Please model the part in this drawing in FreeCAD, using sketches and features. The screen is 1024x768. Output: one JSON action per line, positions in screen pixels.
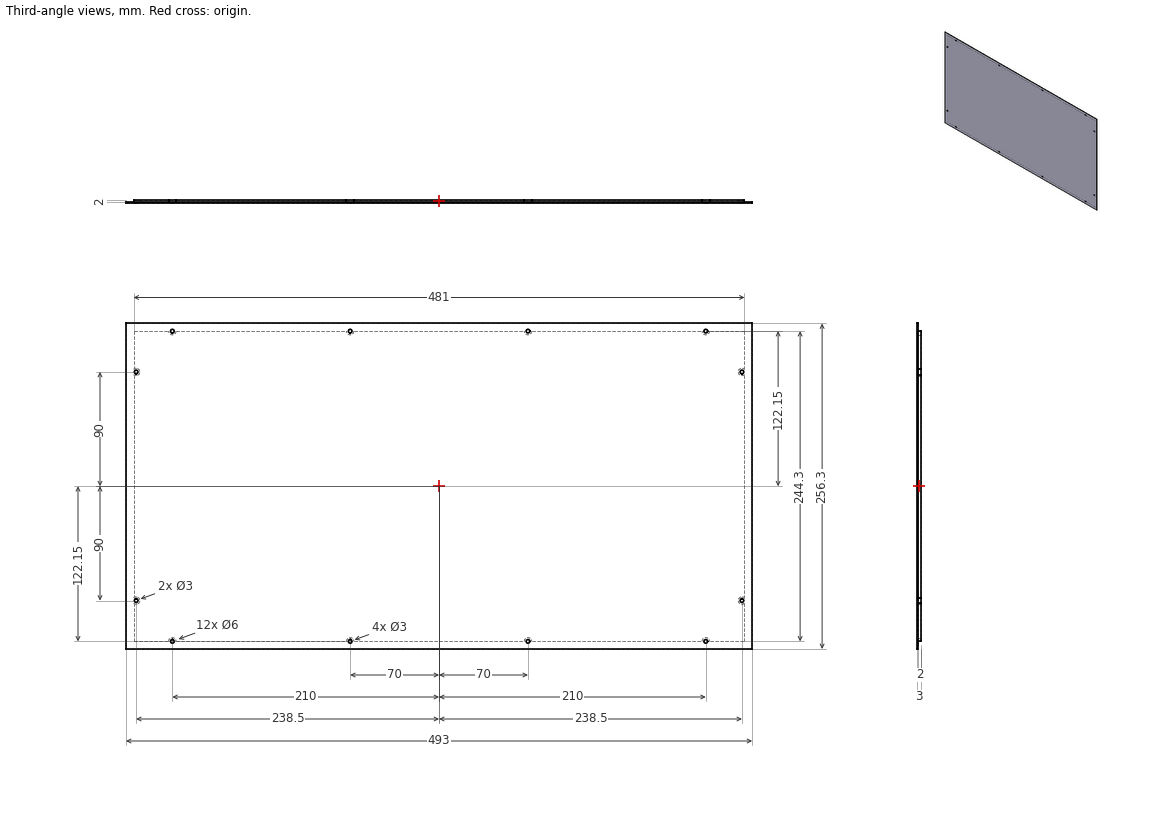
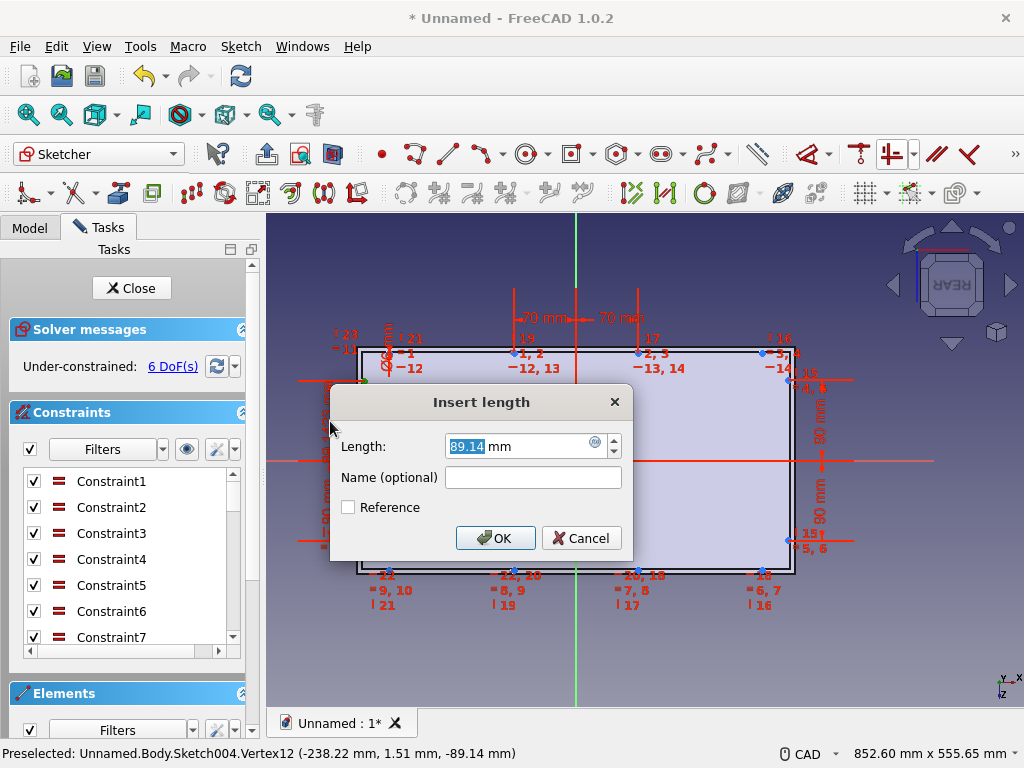
{"action": "type", "text": "90"}
{"action": "key", "text": "Return"}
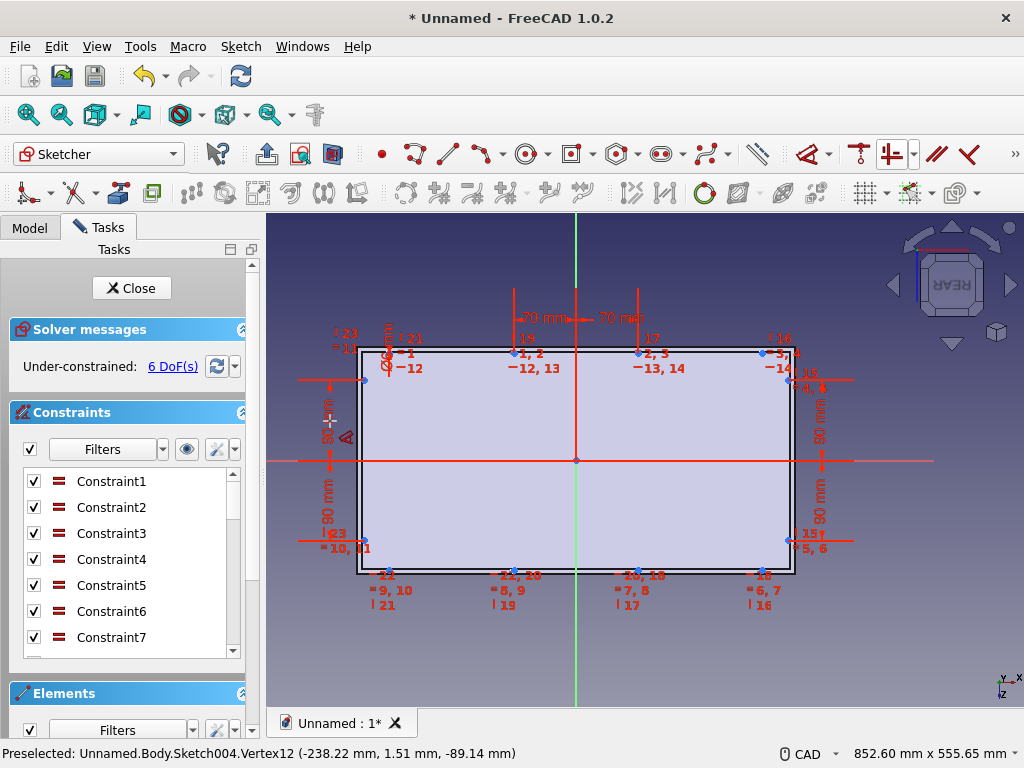
{"action": "left_click", "coordinate": [389, 353]}
{"action": "left_click", "coordinate": [440, 319]}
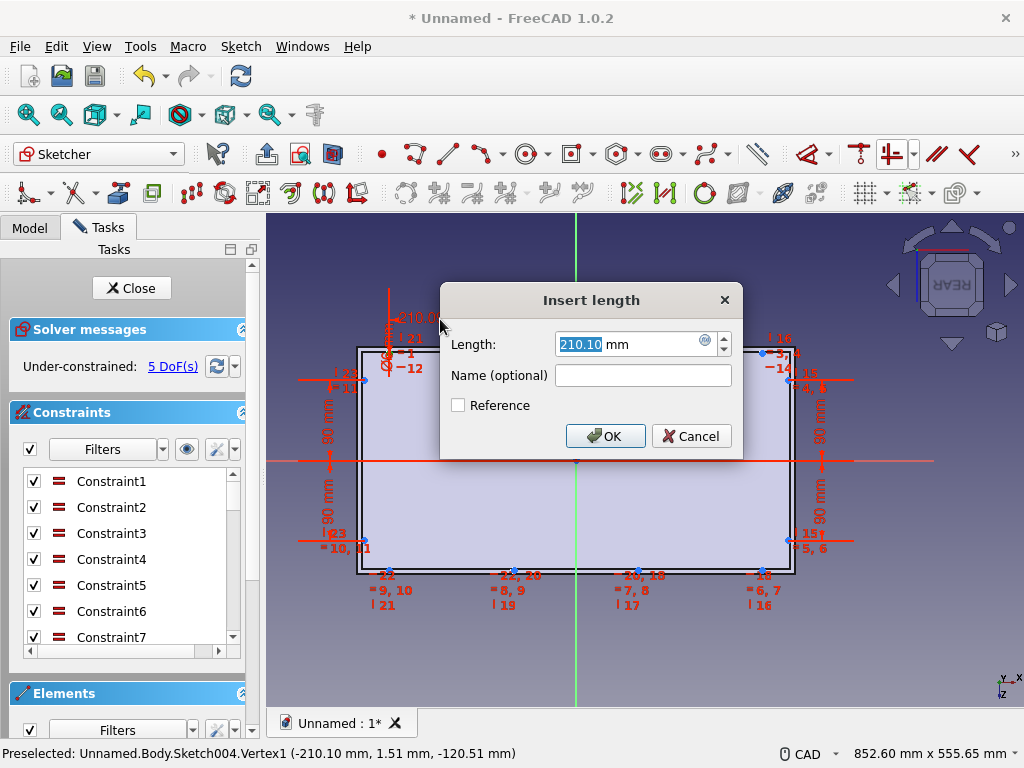
{"action": "type", "text": "210"}
{"action": "key", "text": "Return"}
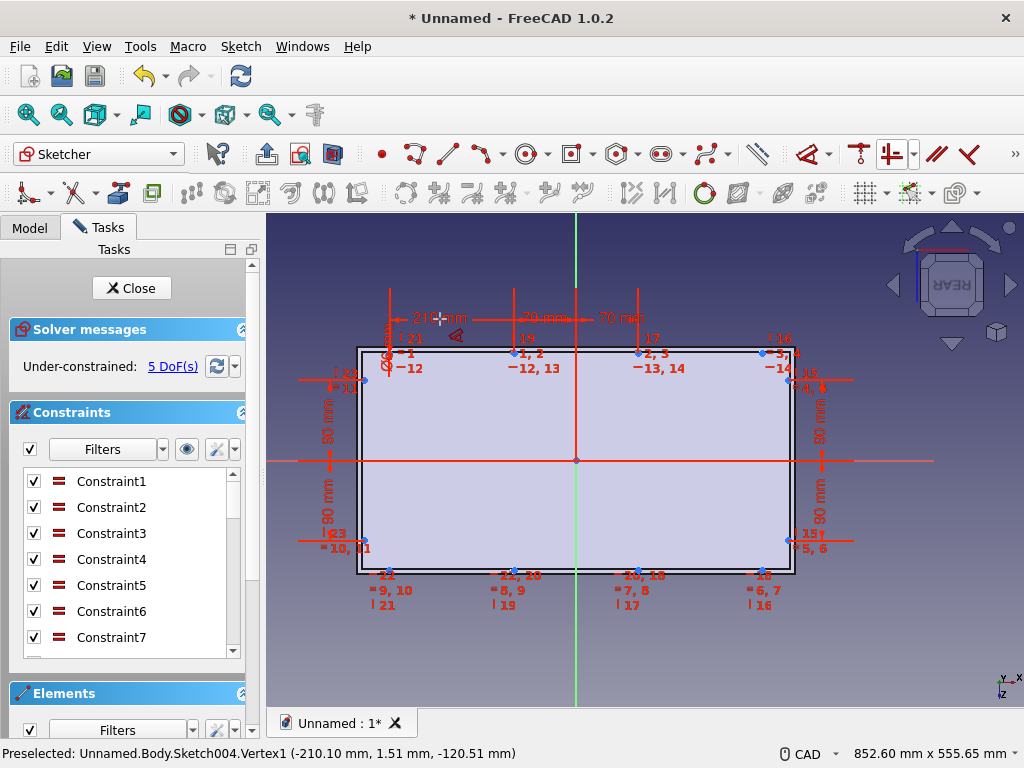
{"action": "left_click", "coordinate": [762, 353]}
{"action": "left_click", "coordinate": [712, 319]}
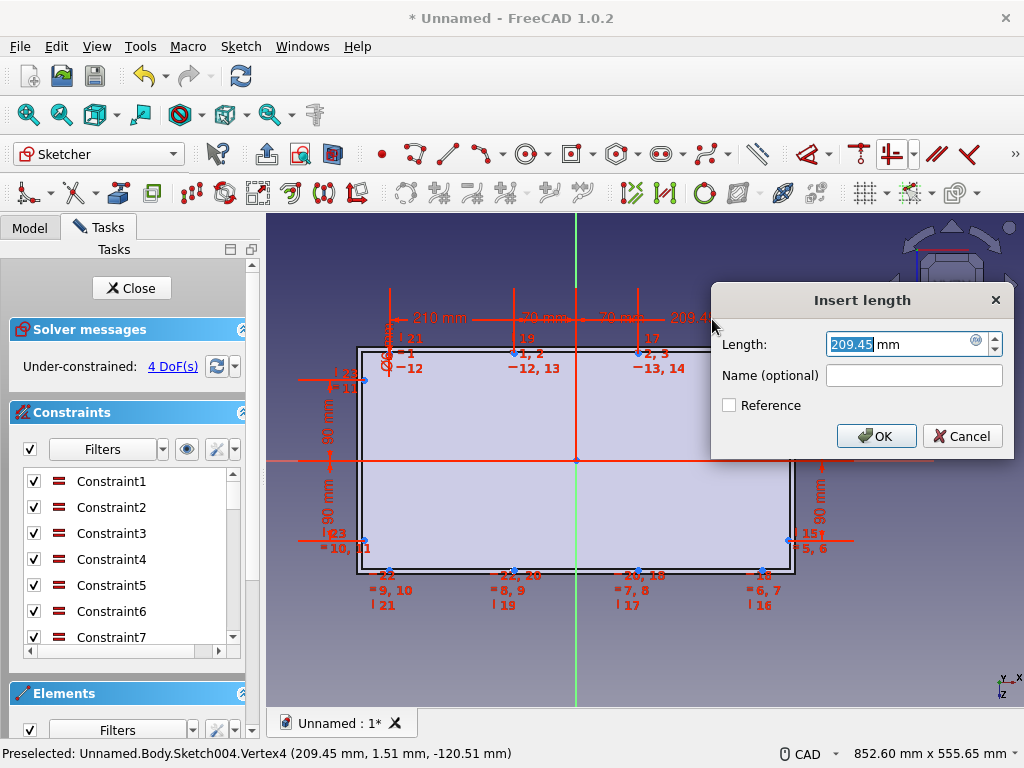
{"action": "type", "text": "210"}
{"action": "key", "text": "Return"}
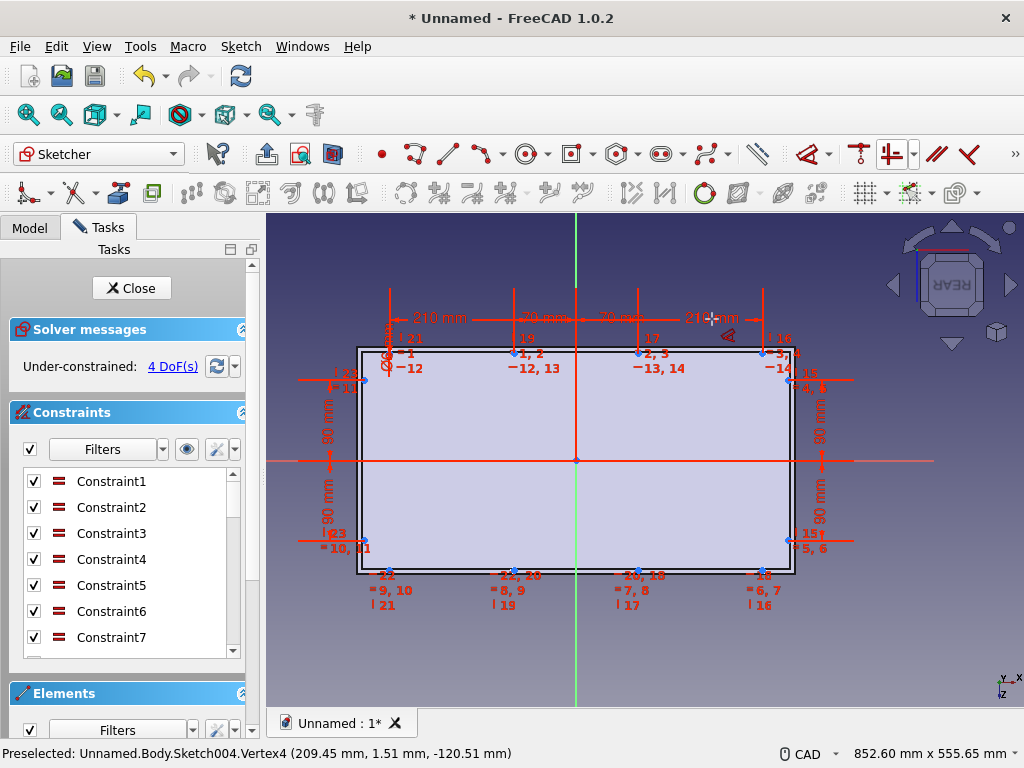
{"action": "left_click", "coordinate": [788, 380]}
{"action": "left_click", "coordinate": [682, 346]}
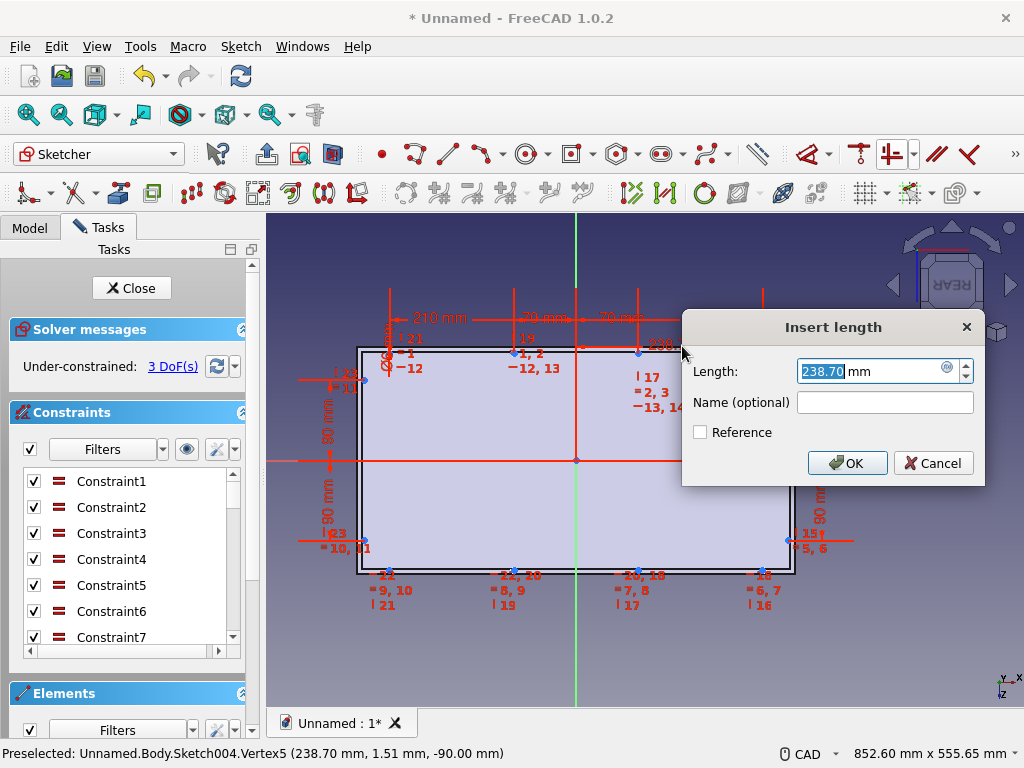
{"action": "type", "text": "238.5"}
{"action": "key", "text": "Return"}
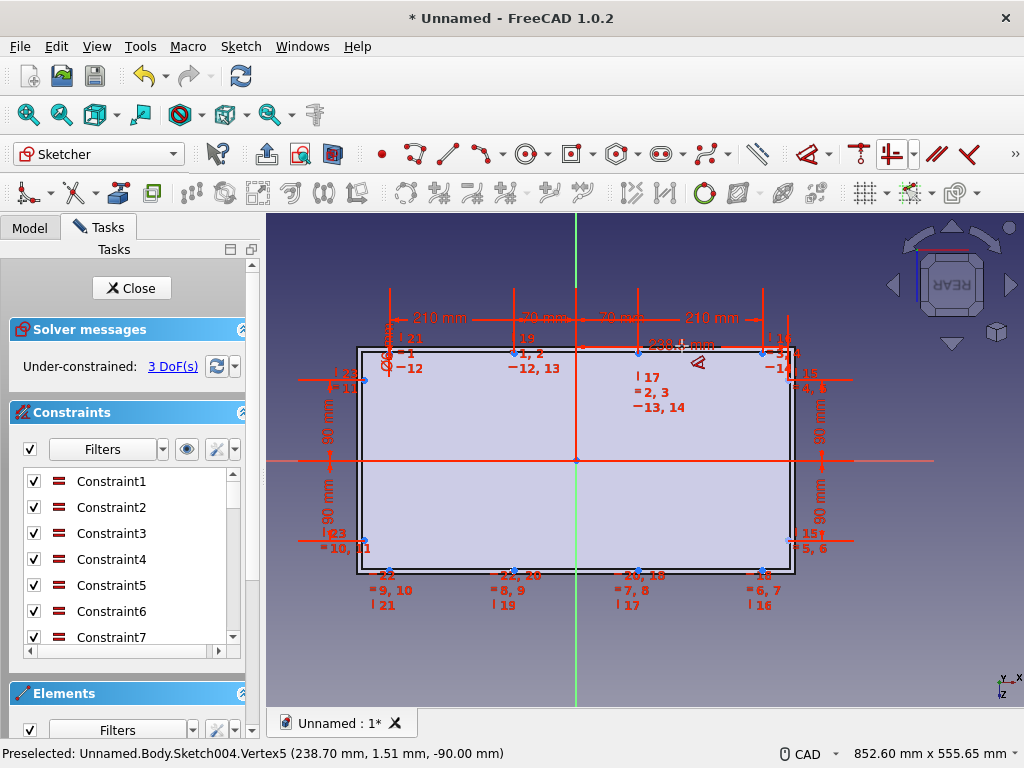
{"action": "left_click", "coordinate": [364, 541]}
{"action": "left_click", "coordinate": [470, 575]}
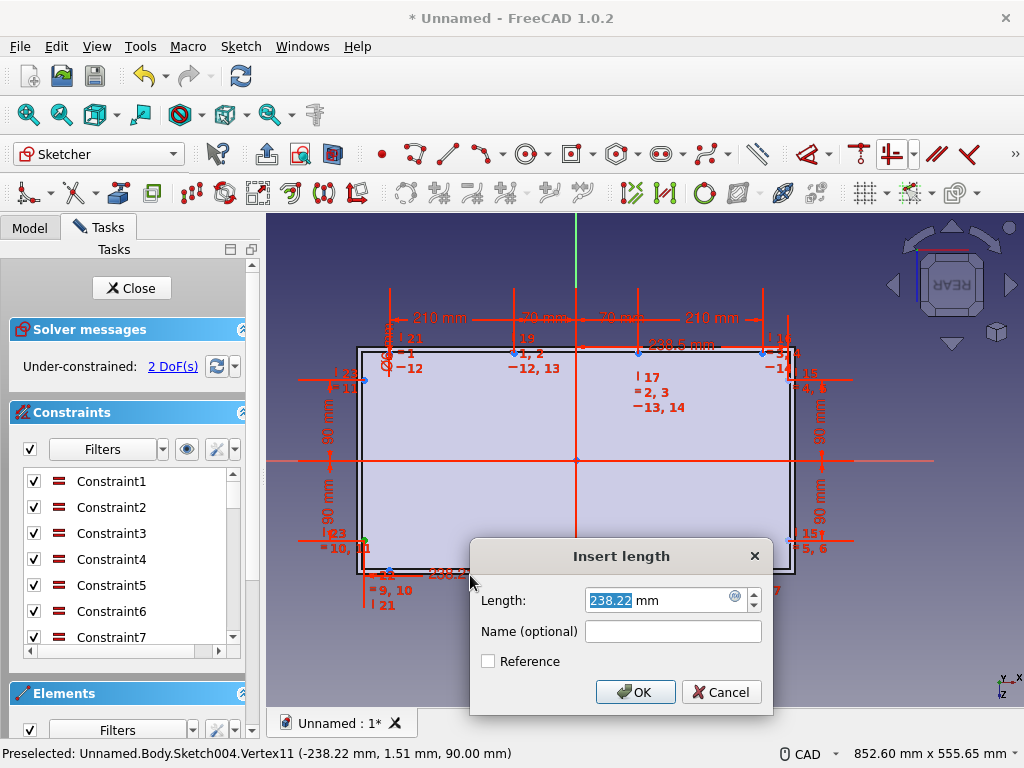
{"action": "type", "text": "238.5"}
{"action": "key", "text": "Return"}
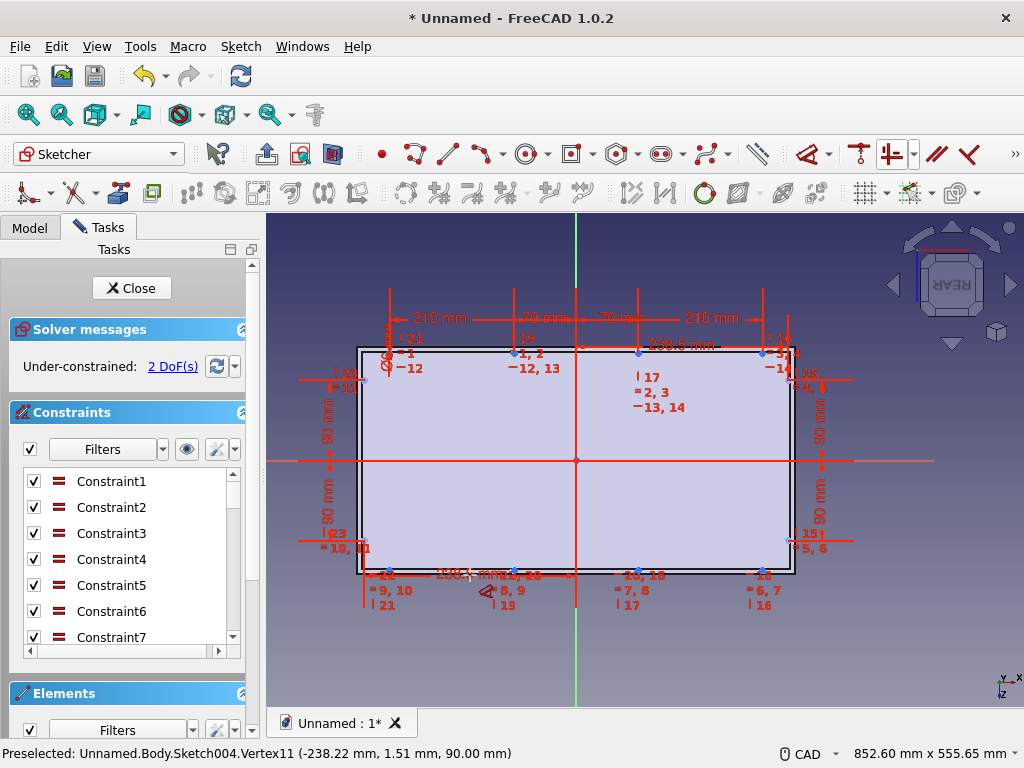
{"action": "left_click", "coordinate": [390, 353]}
{"action": "left_click", "coordinate": [356, 444]}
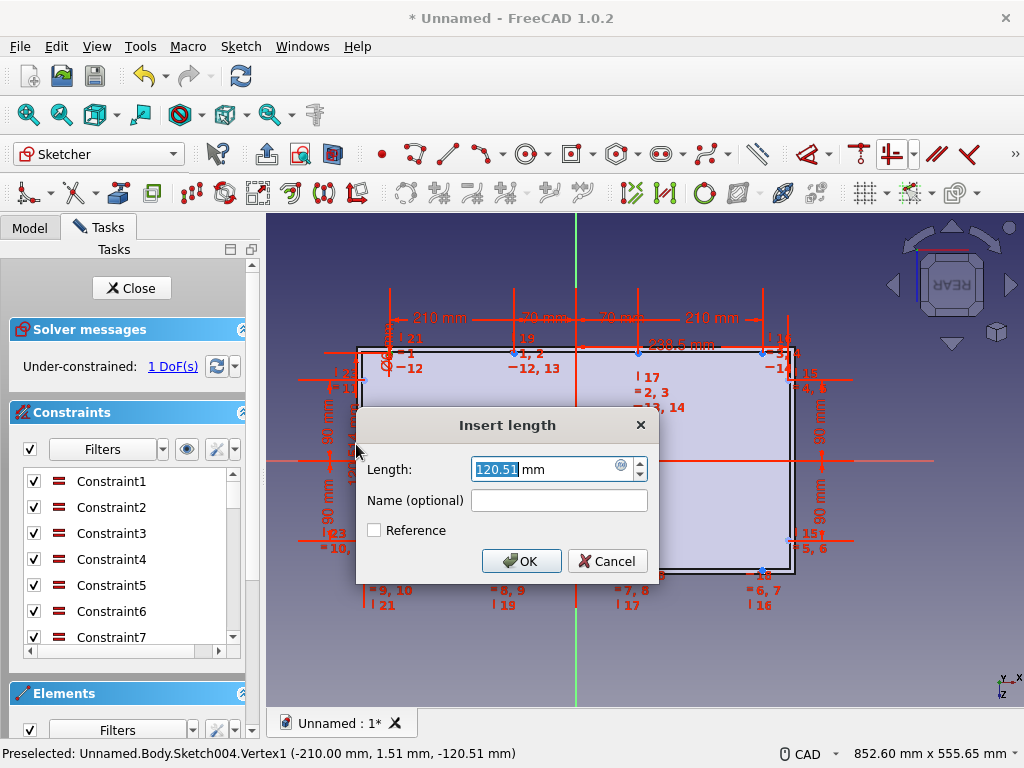
{"action": "type", "text": "122.15"}
{"action": "key", "text": "Return"}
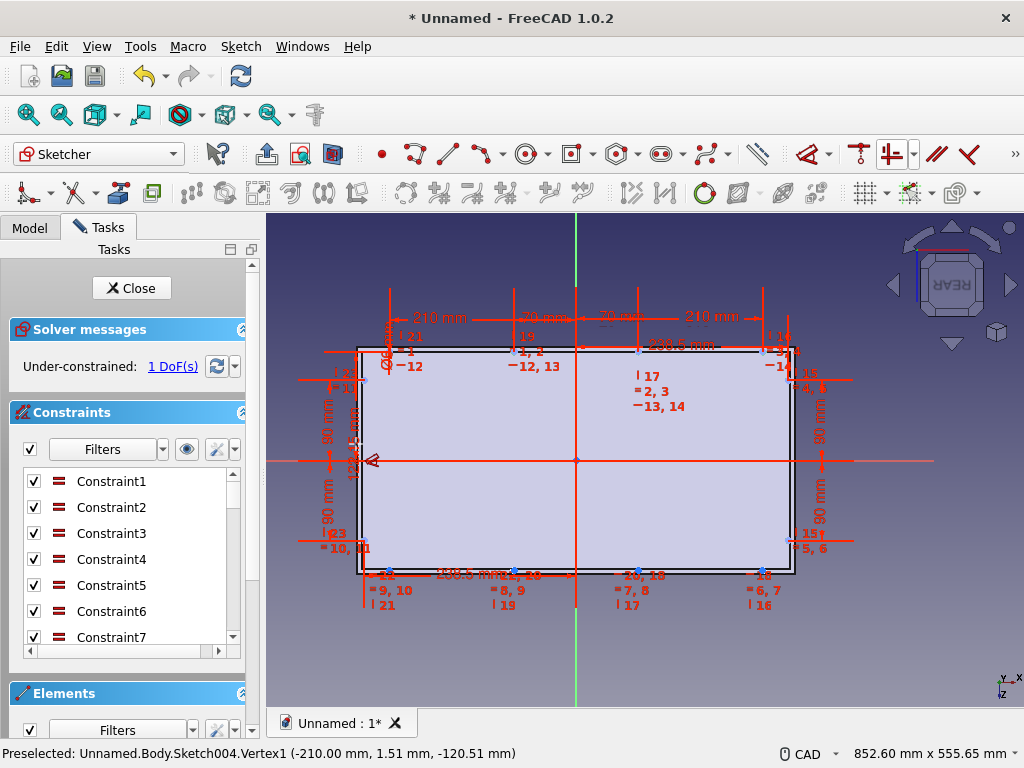
{"action": "left_click", "coordinate": [763, 570]}
{"action": "left_click", "coordinate": [797, 477]}